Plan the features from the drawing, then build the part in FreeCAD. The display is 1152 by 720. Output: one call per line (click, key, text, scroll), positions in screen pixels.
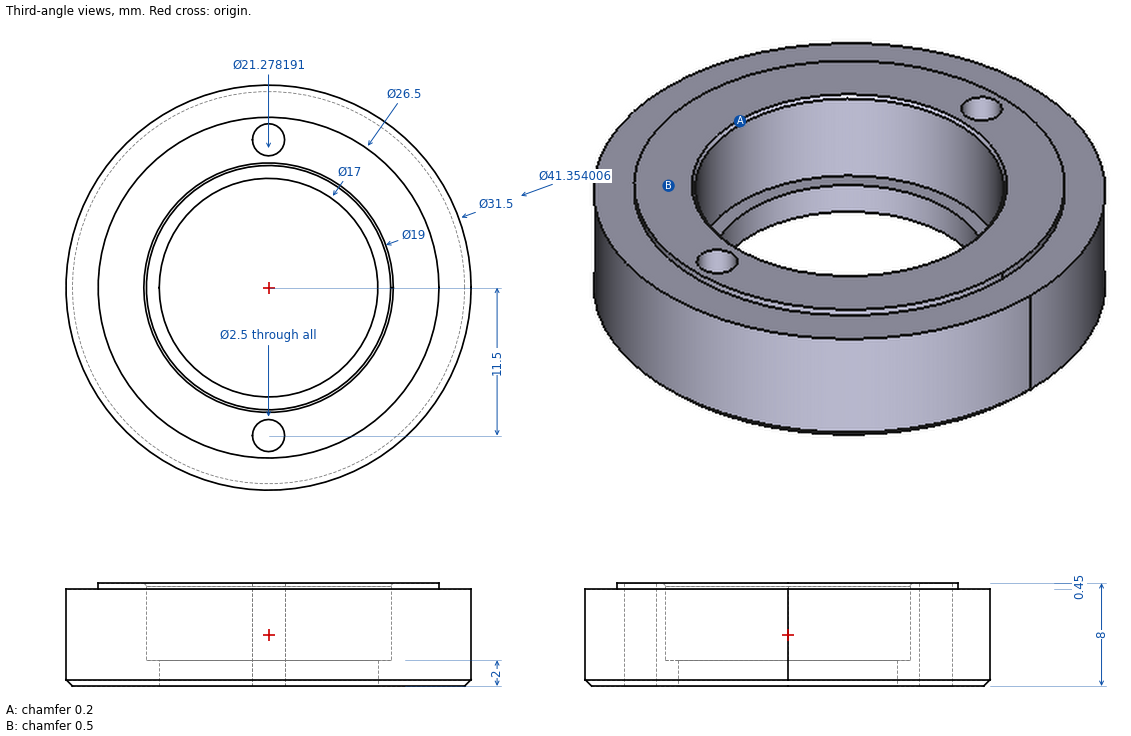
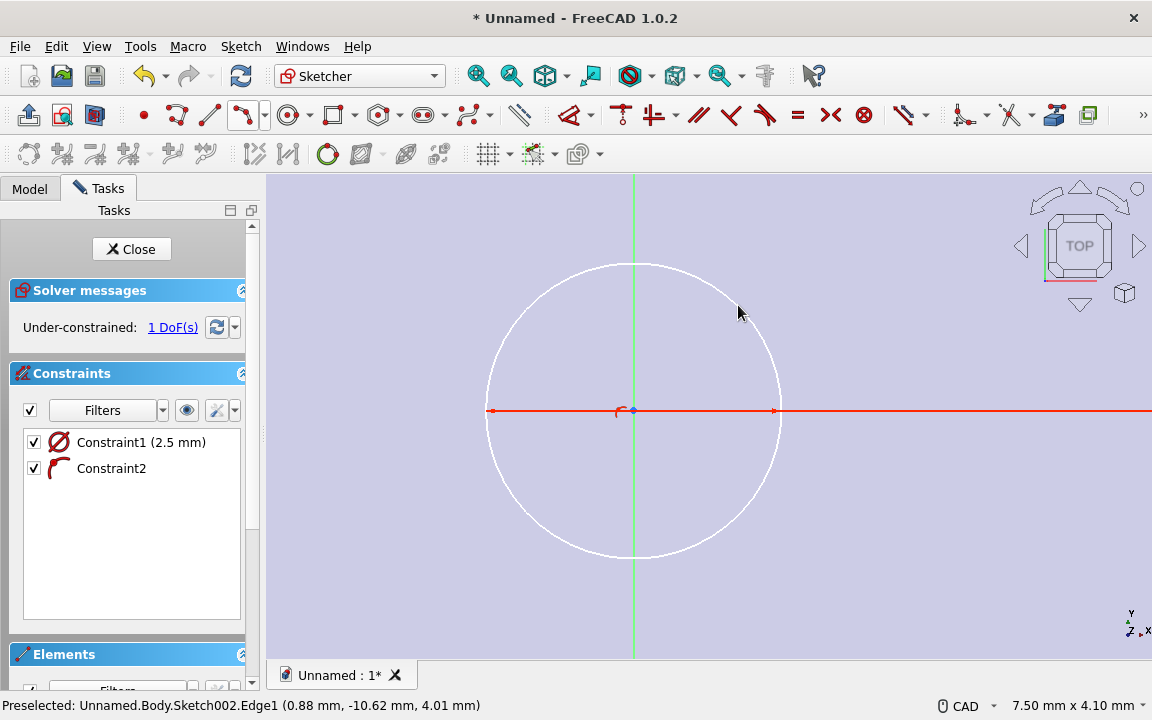
click(634, 411)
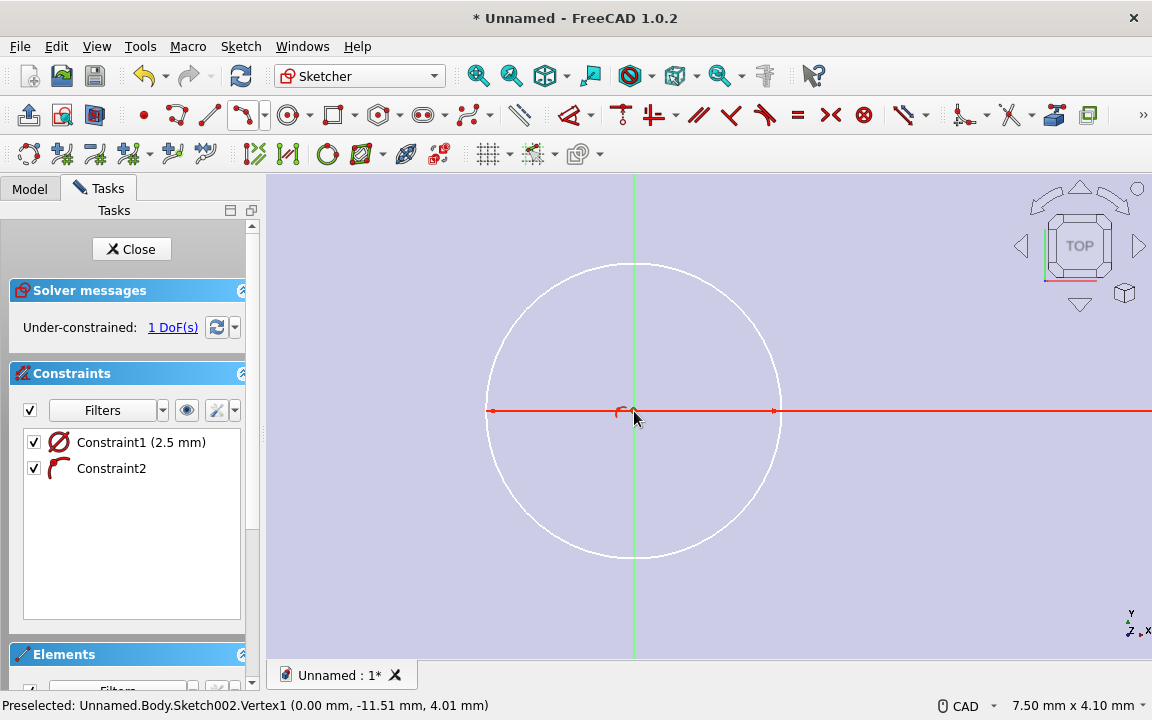
click(590, 116)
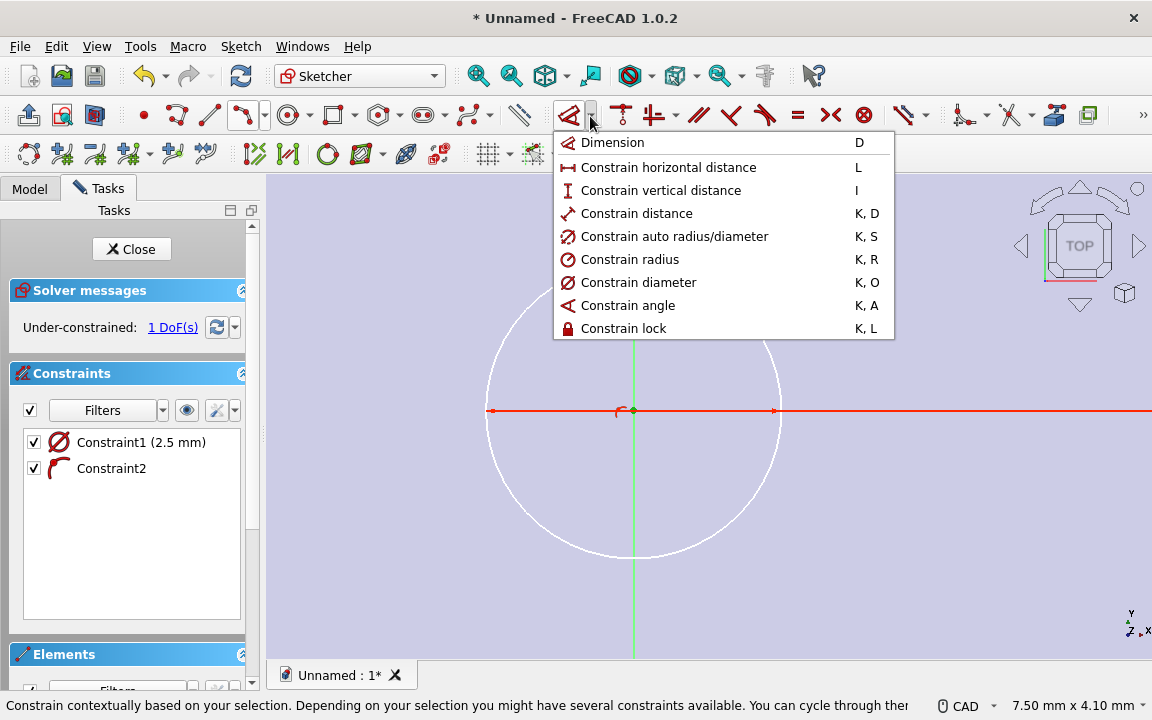
click(724, 190)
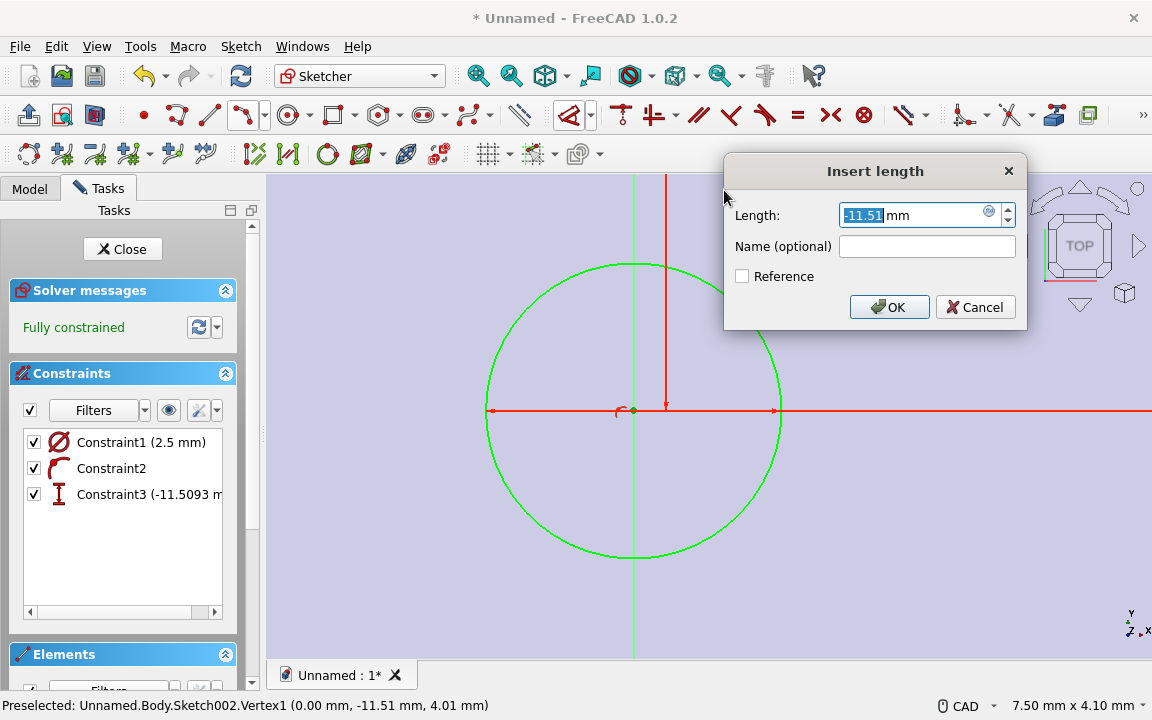
text(-11.5)
key(Return)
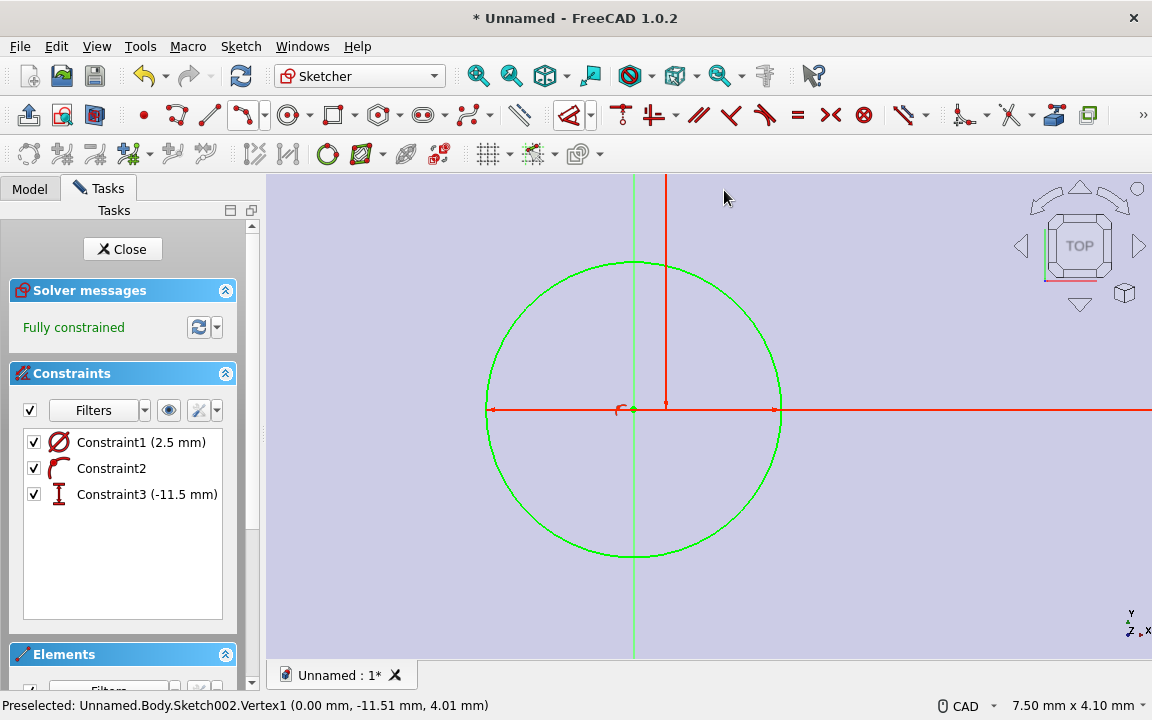
click(123, 249)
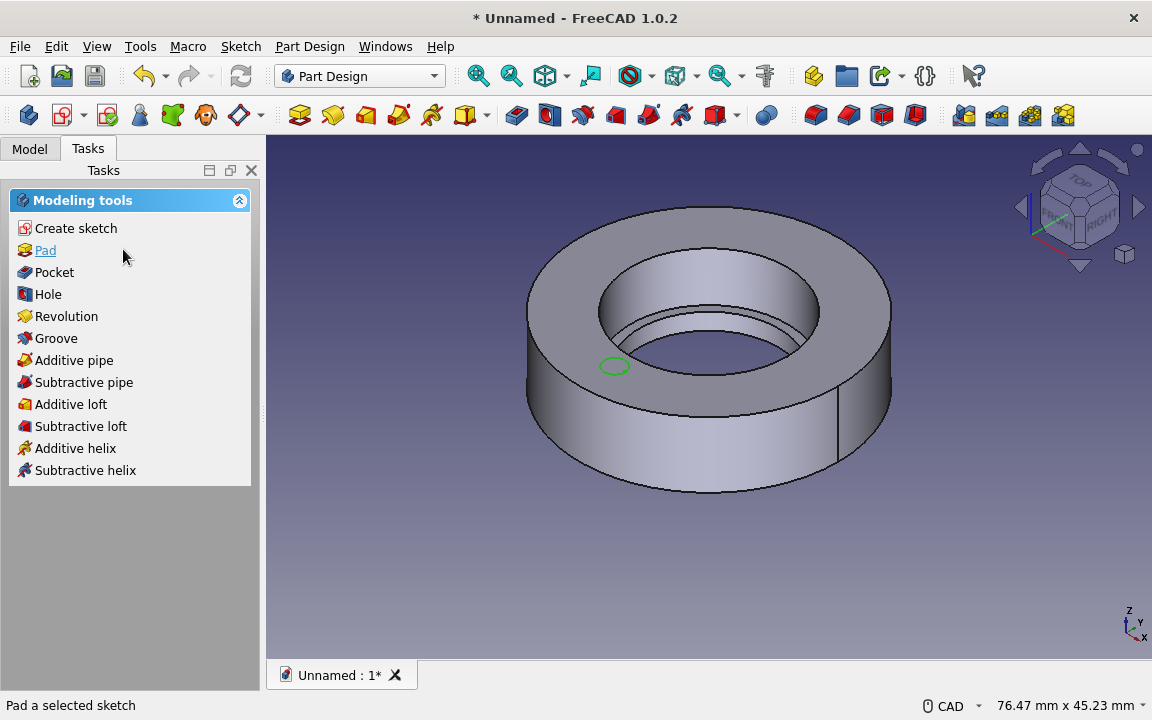
click(550, 116)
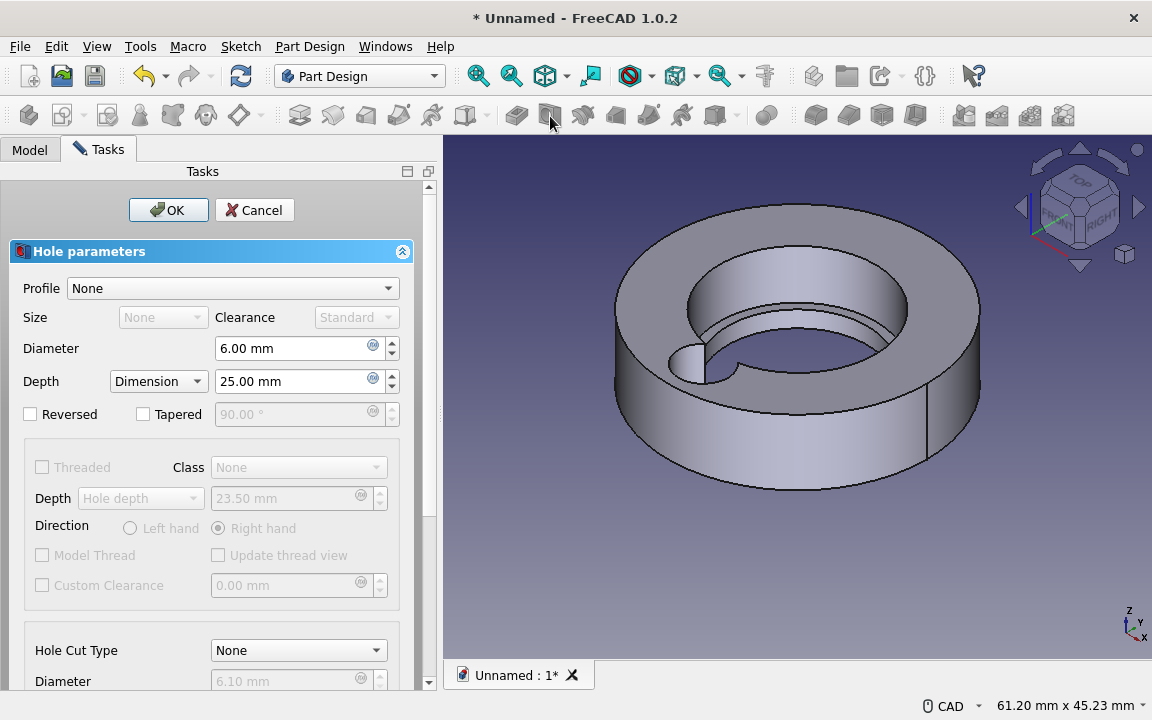
triple_click(300, 348)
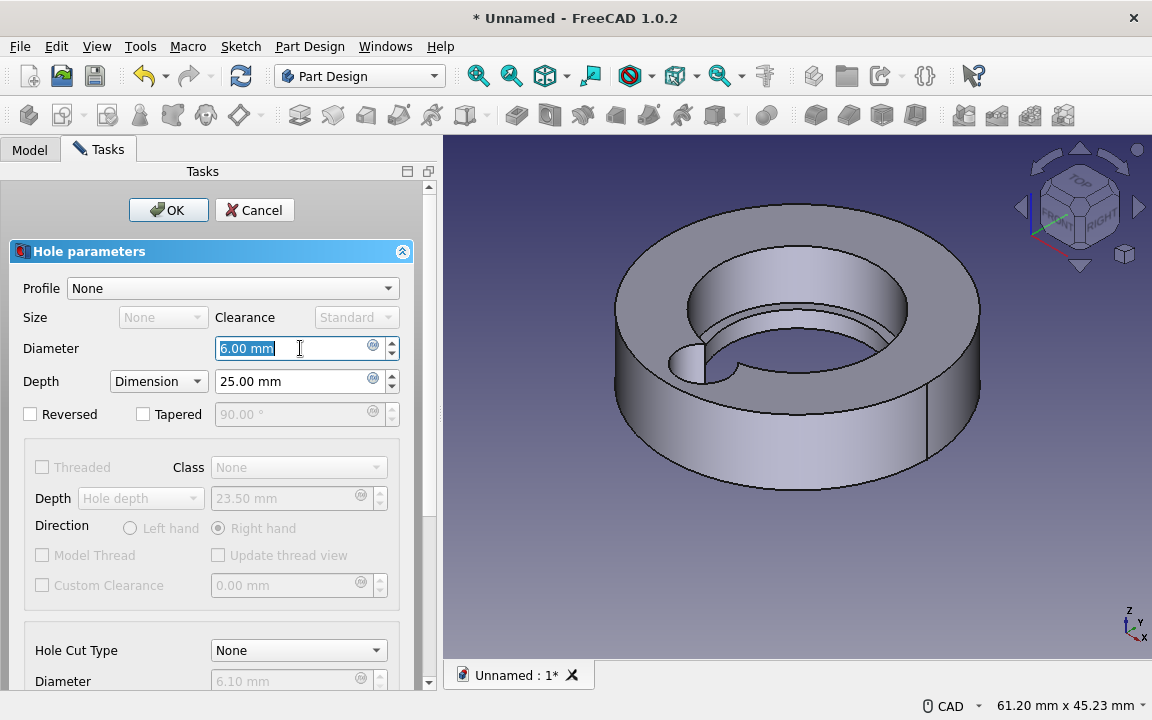
text(2.5)
key(Tab)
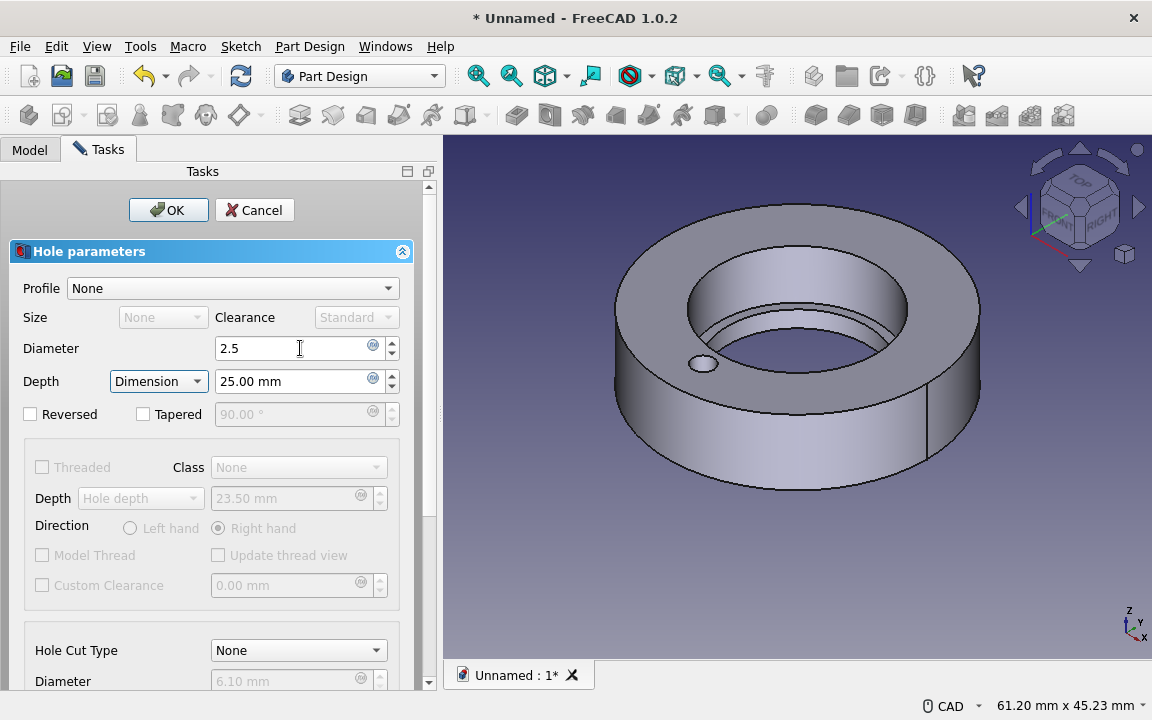
click(160, 382)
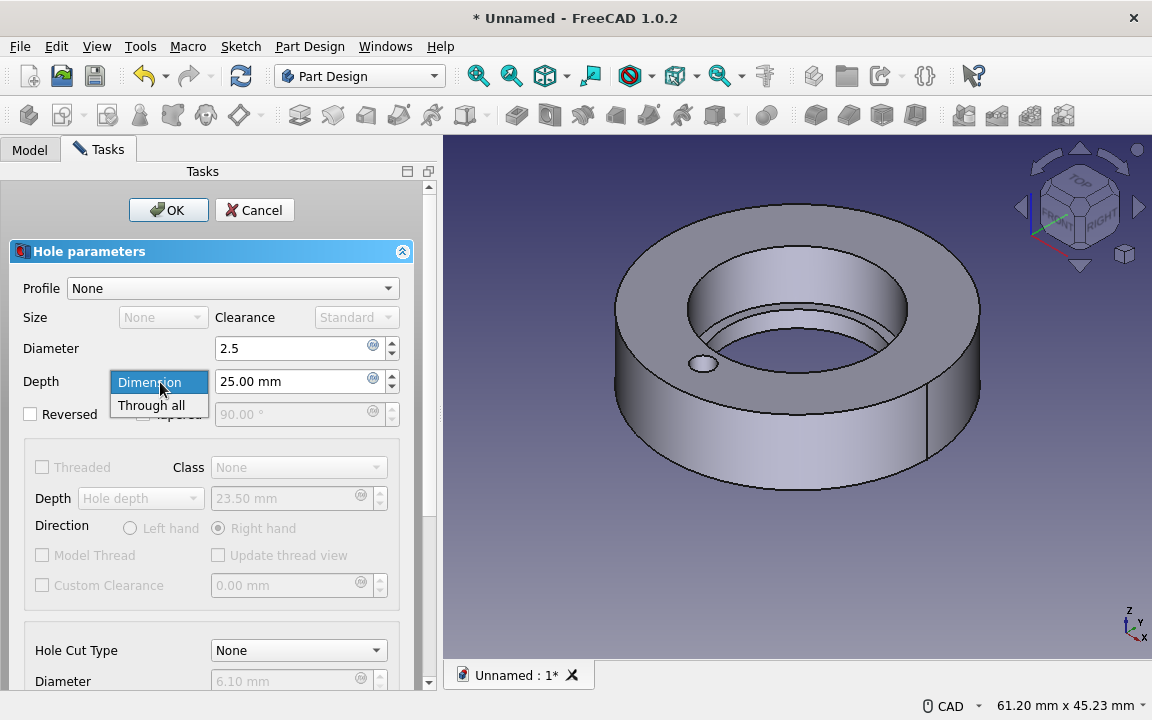
click(158, 406)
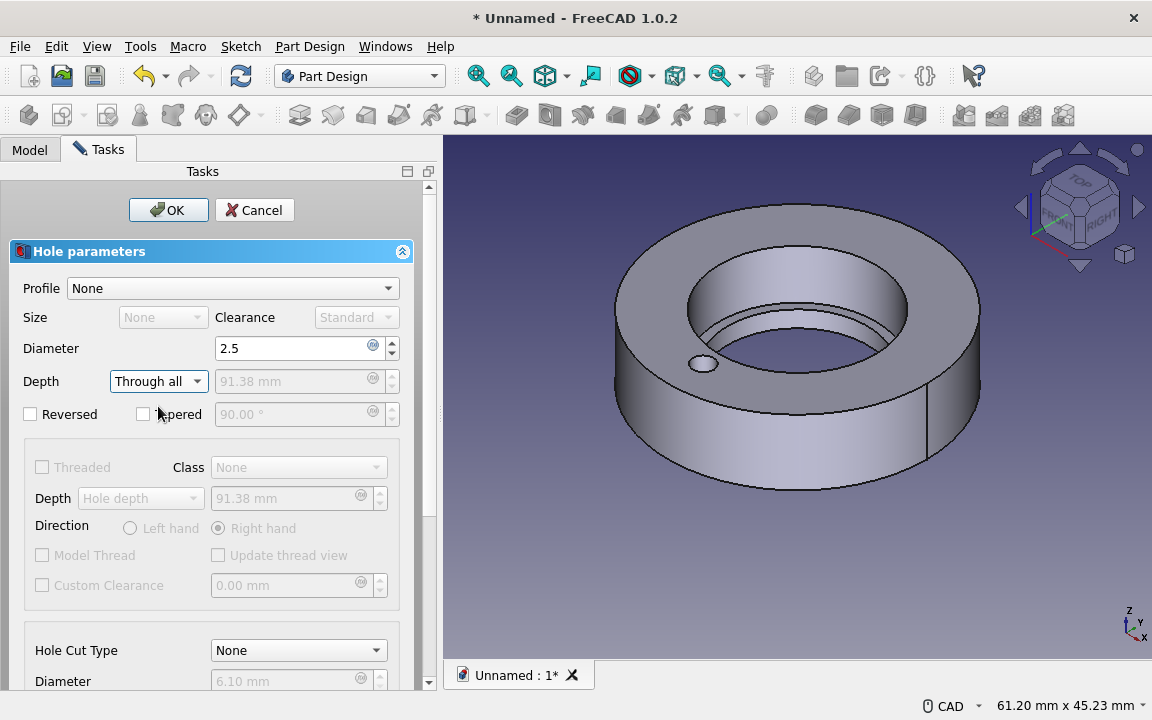
click(169, 210)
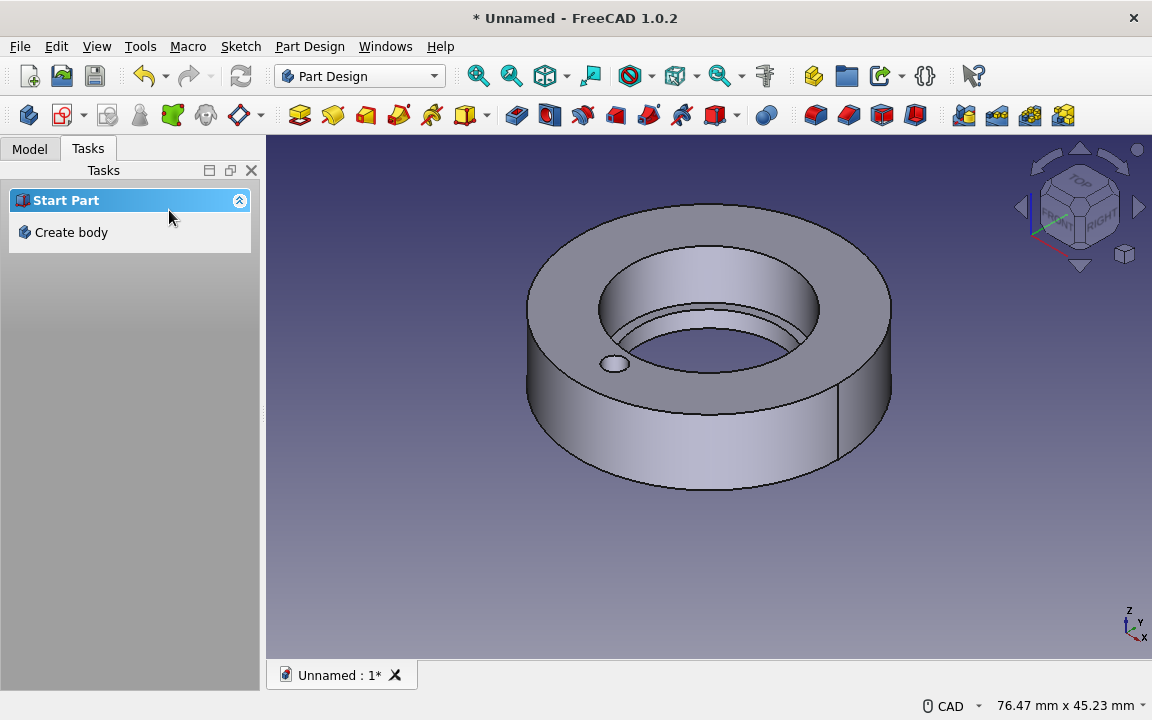
click(30, 148)